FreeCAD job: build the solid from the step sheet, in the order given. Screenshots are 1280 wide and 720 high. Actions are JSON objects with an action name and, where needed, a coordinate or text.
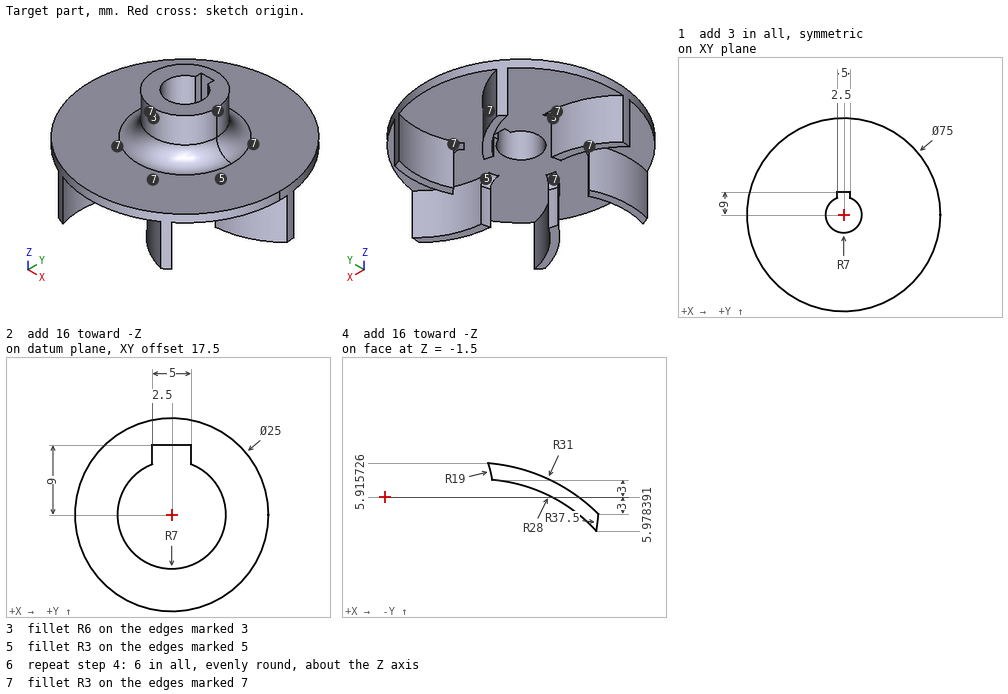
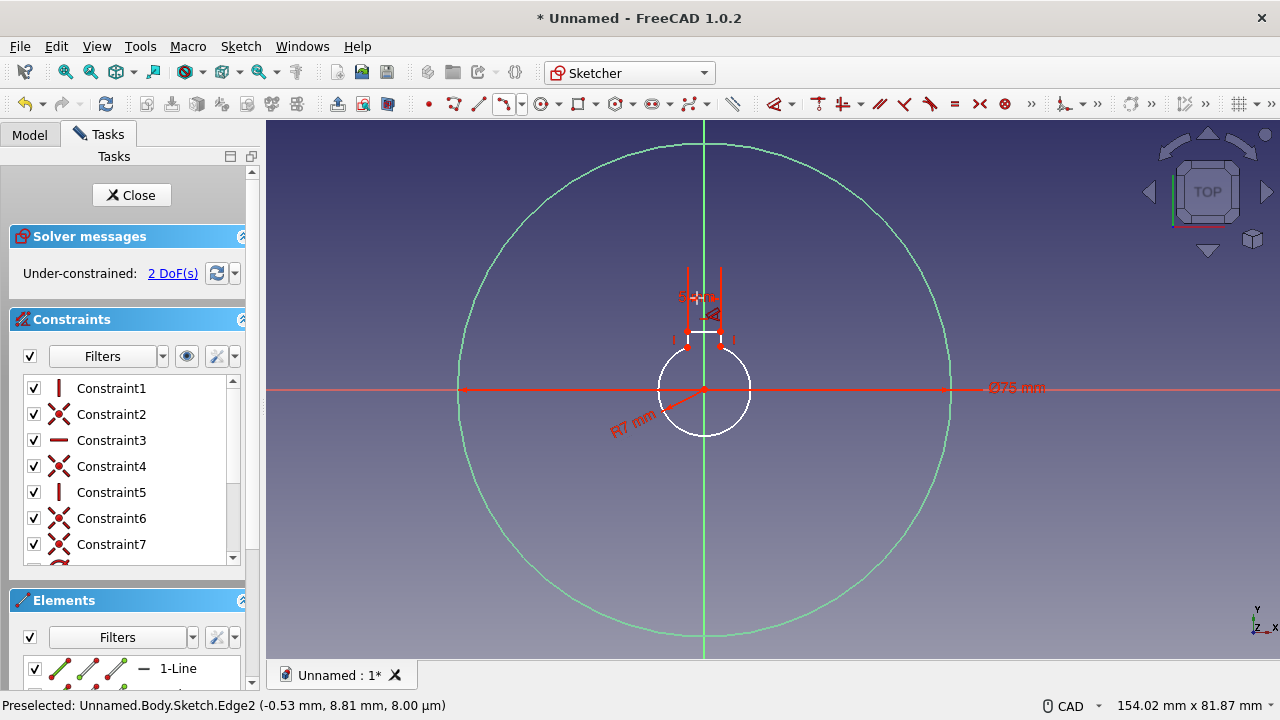
{"action": "left_click", "coordinate": [688, 332]}
{"action": "left_click", "coordinate": [654, 348]}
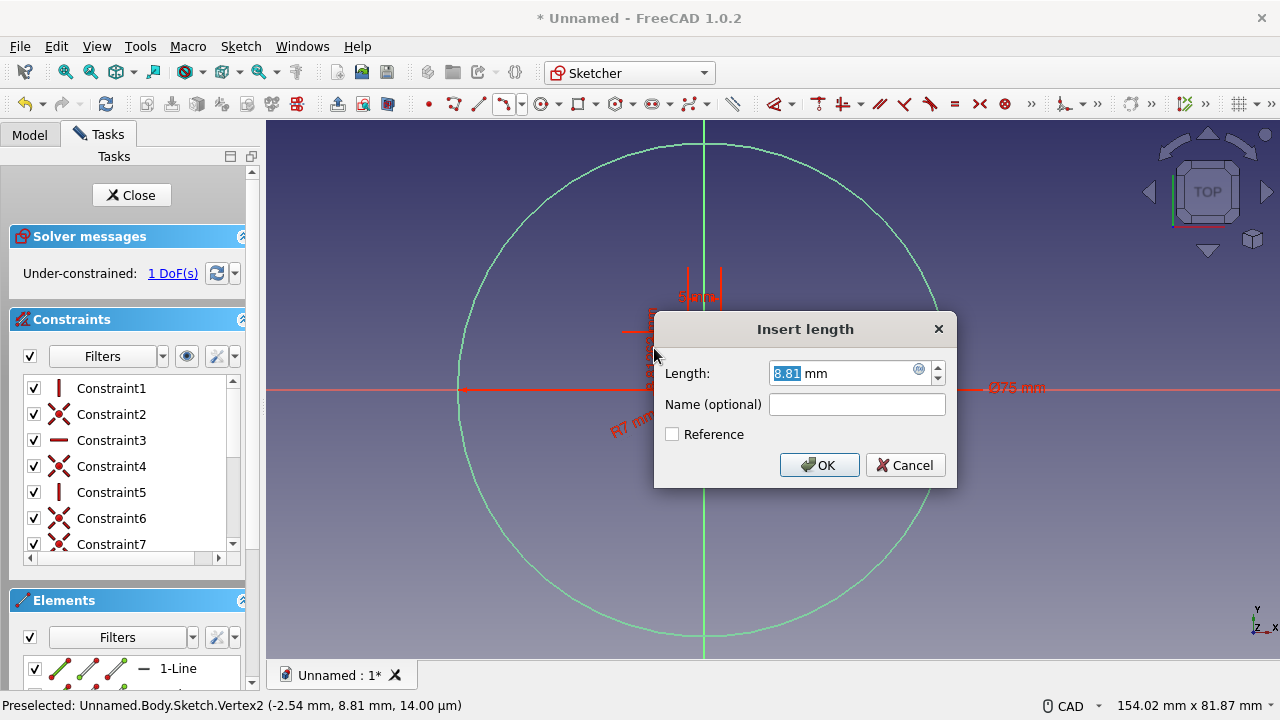
{"action": "type", "text": "9"}
{"action": "key", "text": "Return"}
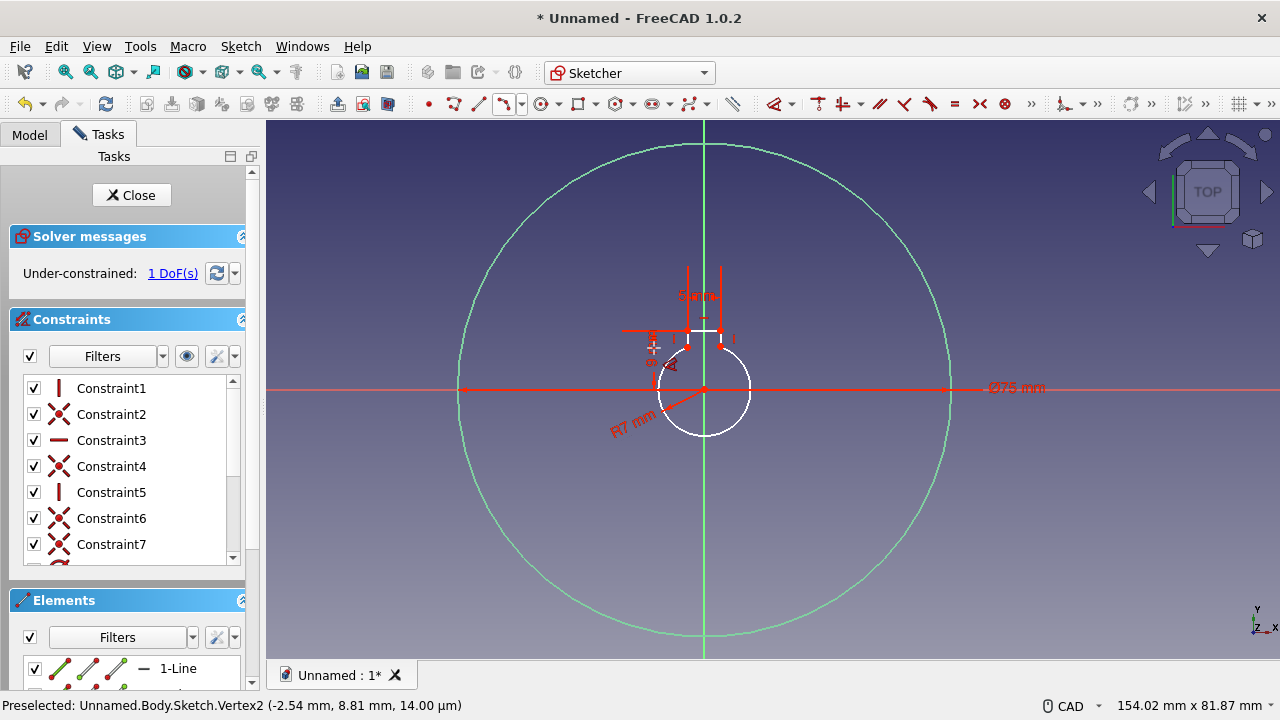
{"action": "scroll", "coordinate": [688, 347], "scroll_direction": "up", "scroll_amount": 5}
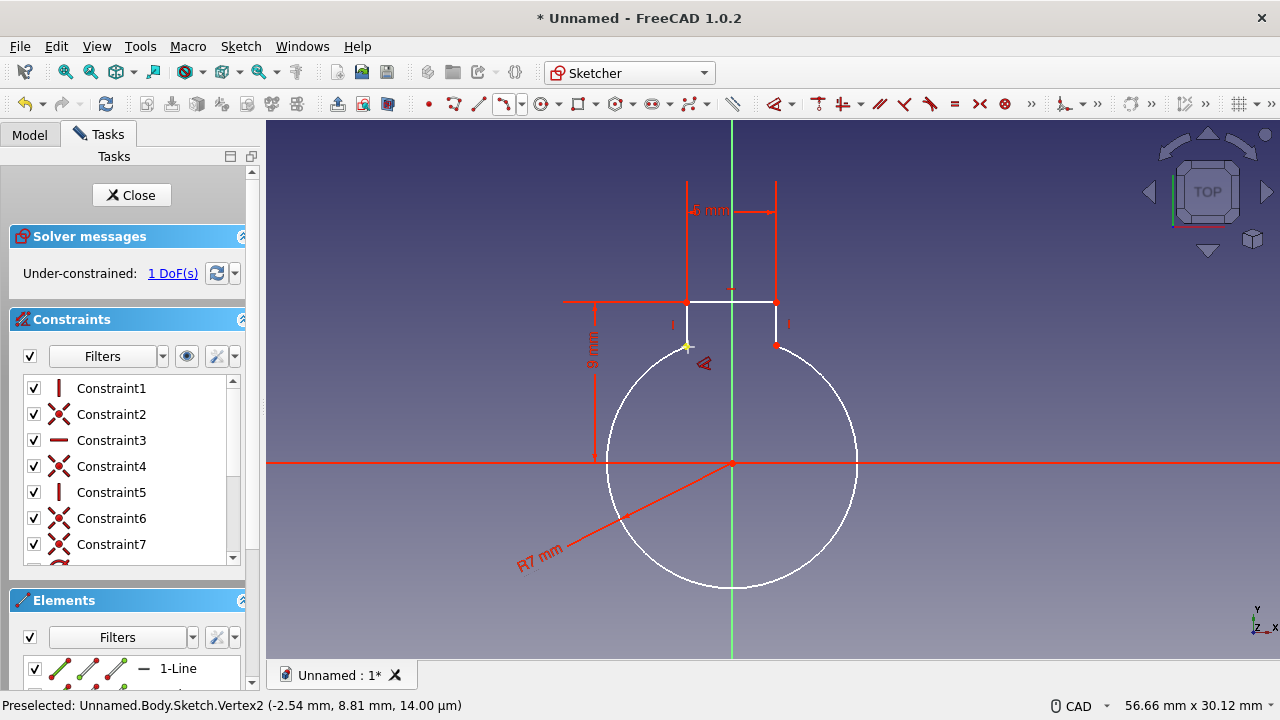
{"action": "left_click", "coordinate": [687, 346]}
{"action": "left_click", "coordinate": [709, 497]}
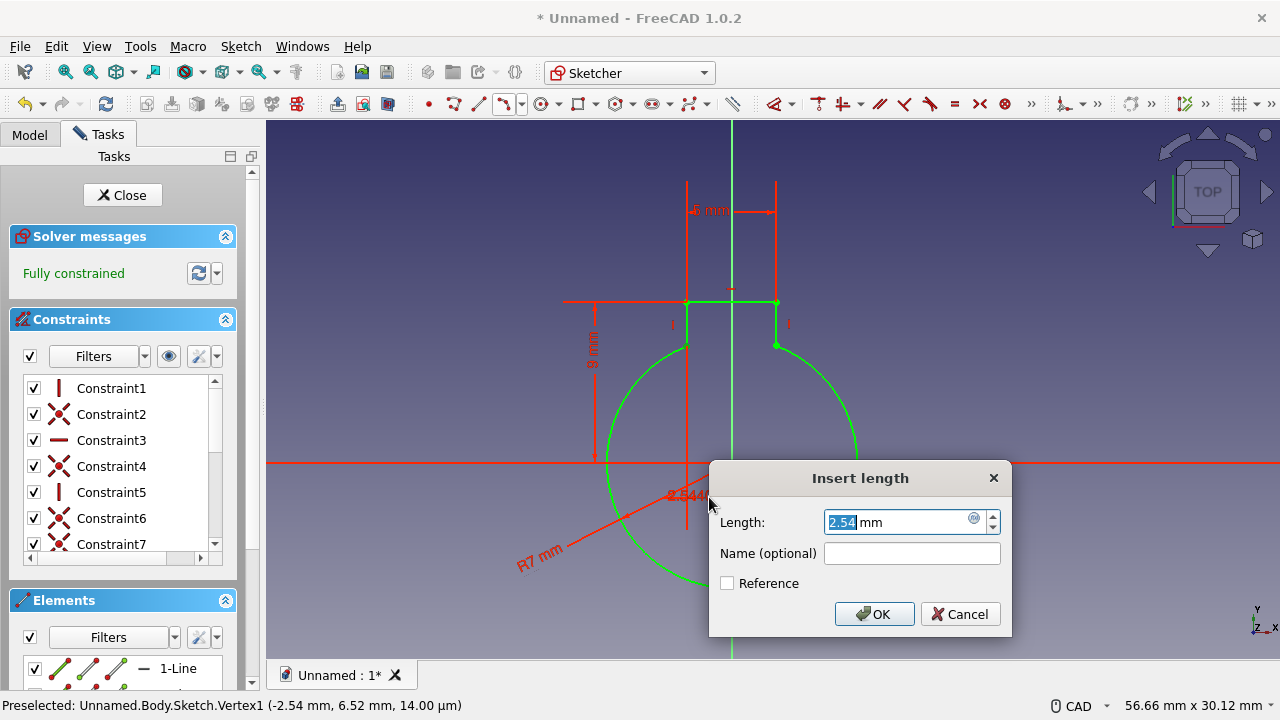
{"action": "type", "text": "2.5"}
{"action": "key", "text": "Return"}
{"action": "key", "text": "Escape"}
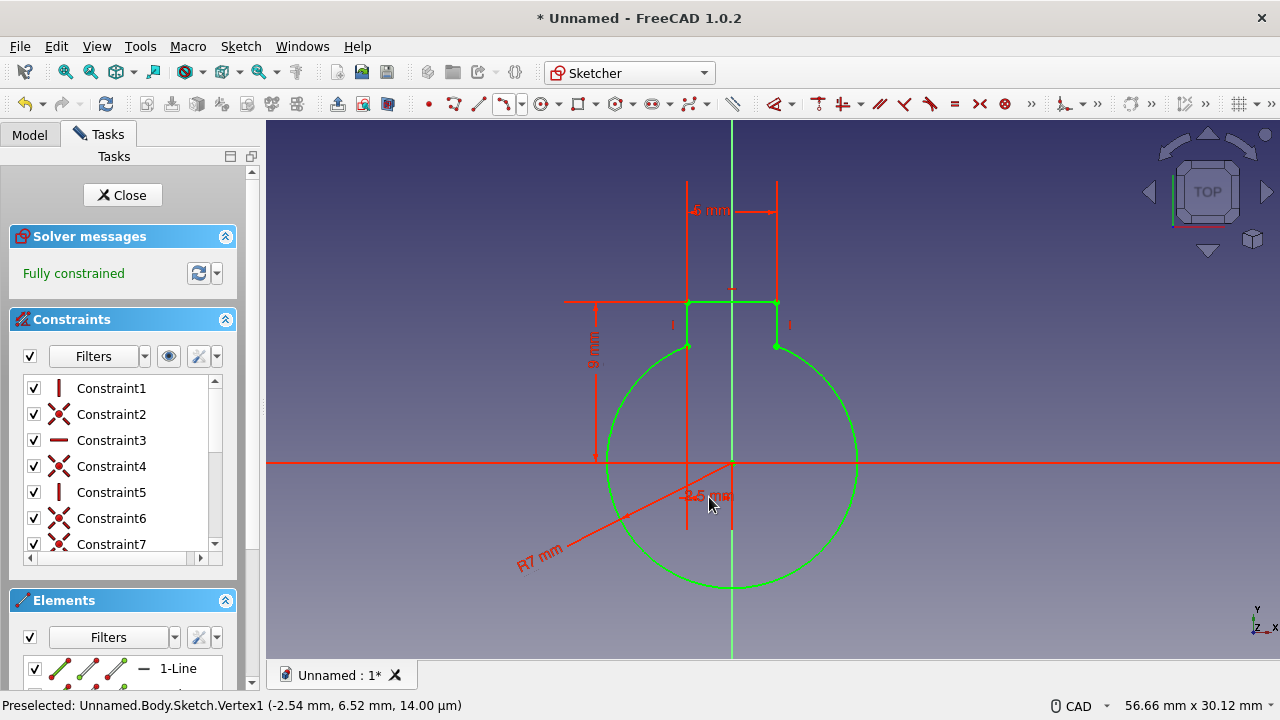
{"action": "left_click", "coordinate": [123, 195]}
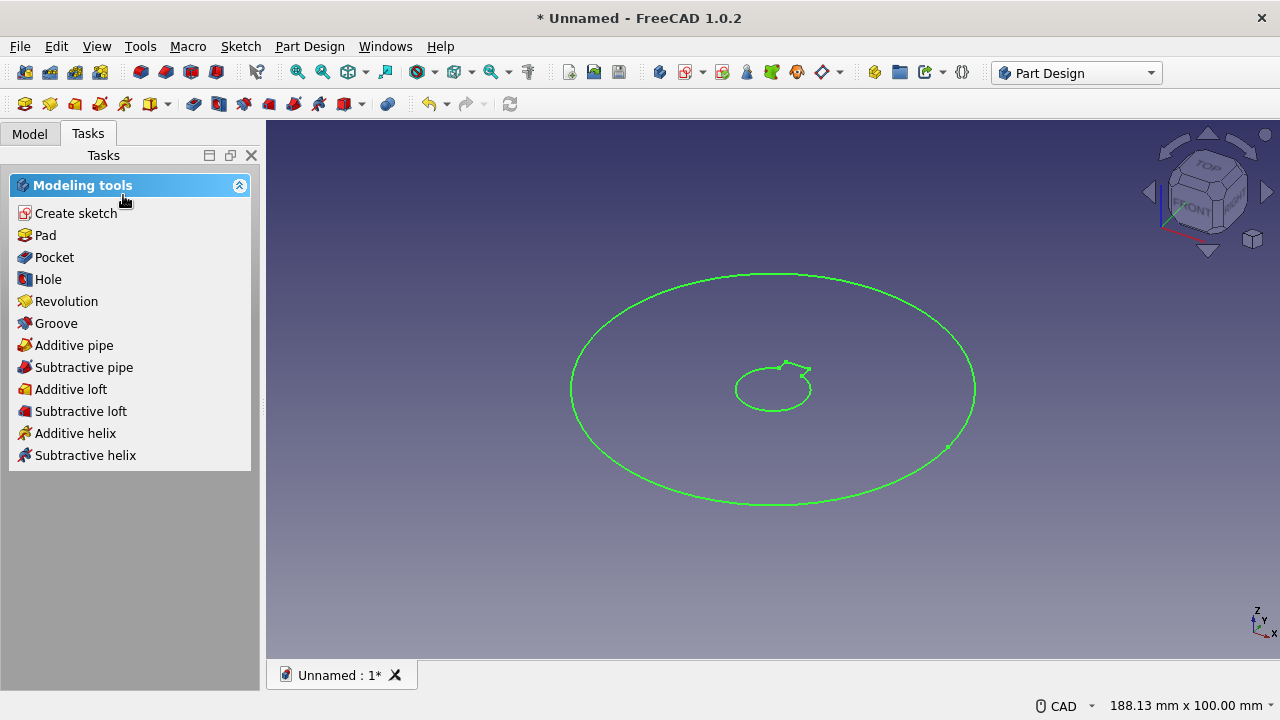
{"action": "left_click", "coordinate": [25, 104]}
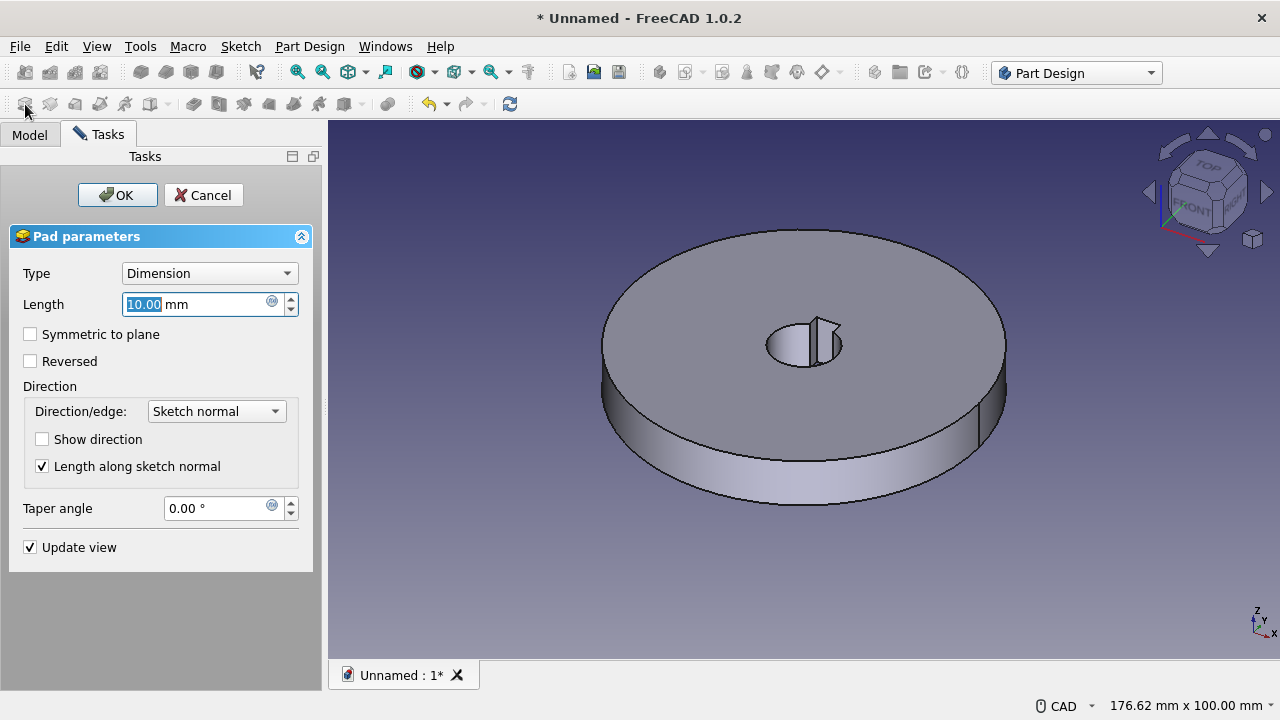
{"action": "type", "text": "3"}
{"action": "key", "text": "Tab"}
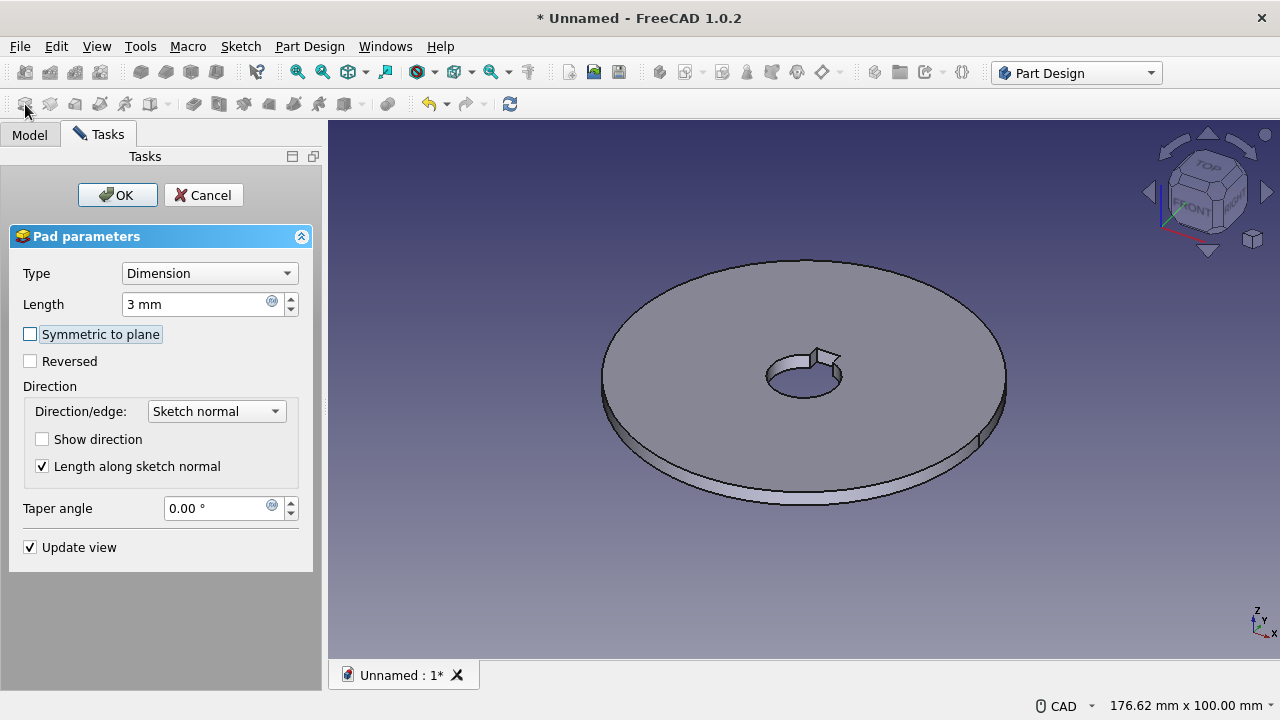
{"action": "left_click", "coordinate": [31, 334]}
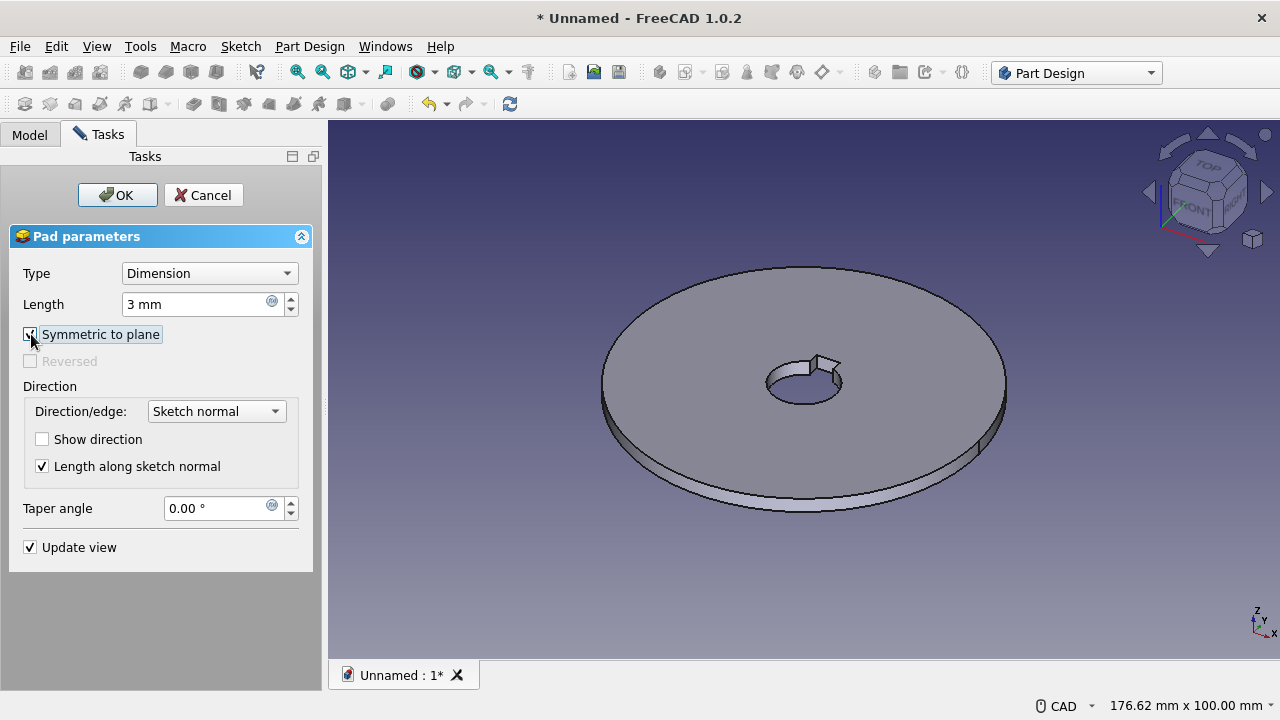
{"action": "left_click", "coordinate": [118, 195]}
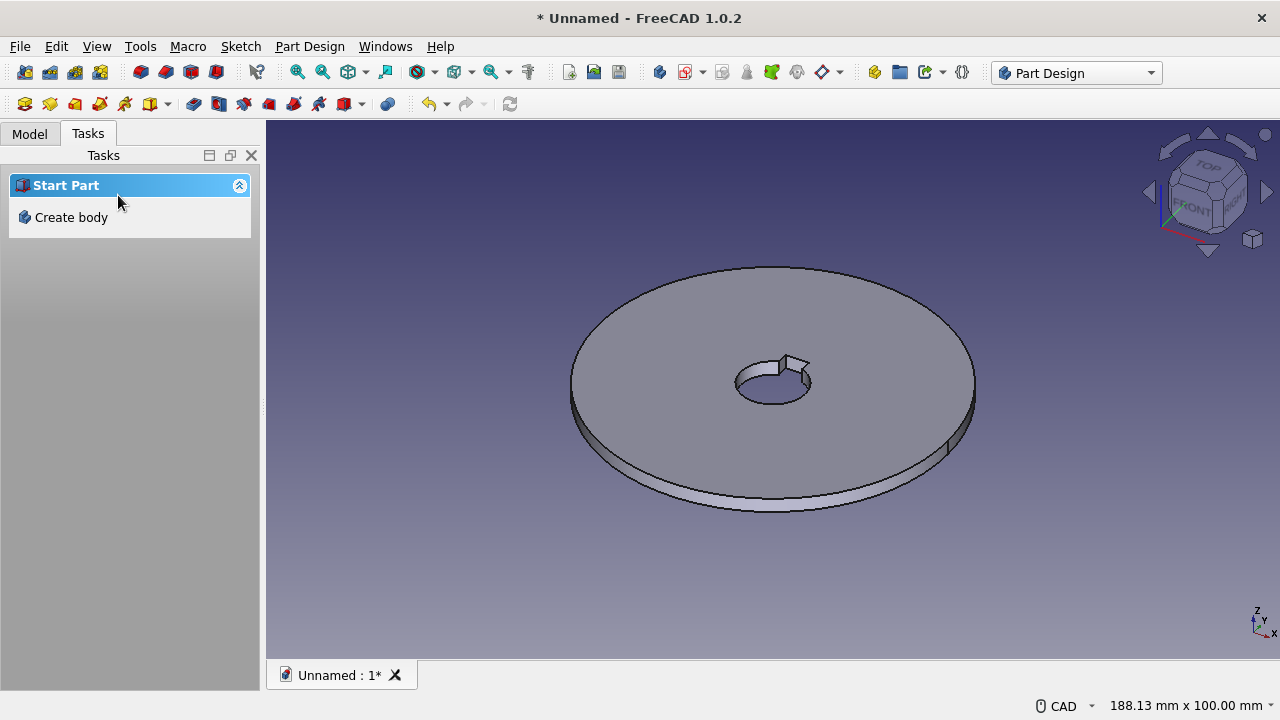
{"action": "left_click", "coordinate": [30, 134]}